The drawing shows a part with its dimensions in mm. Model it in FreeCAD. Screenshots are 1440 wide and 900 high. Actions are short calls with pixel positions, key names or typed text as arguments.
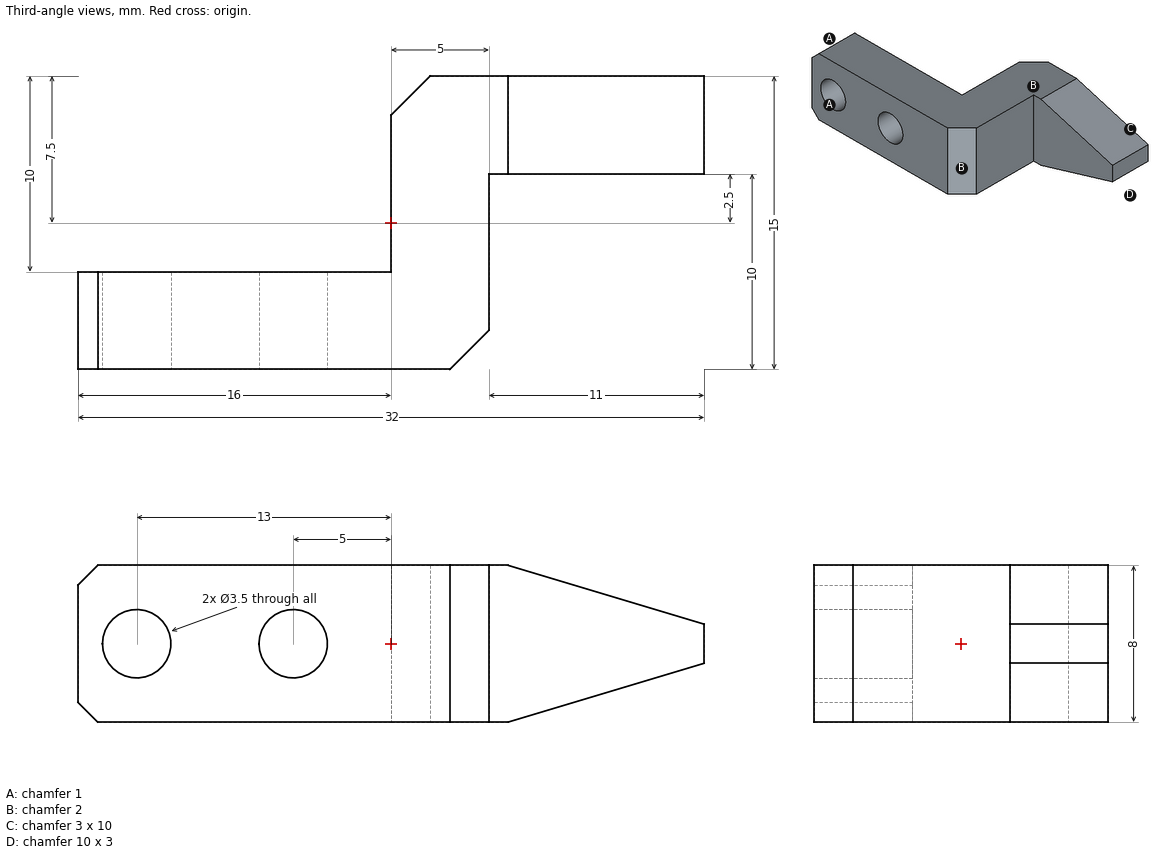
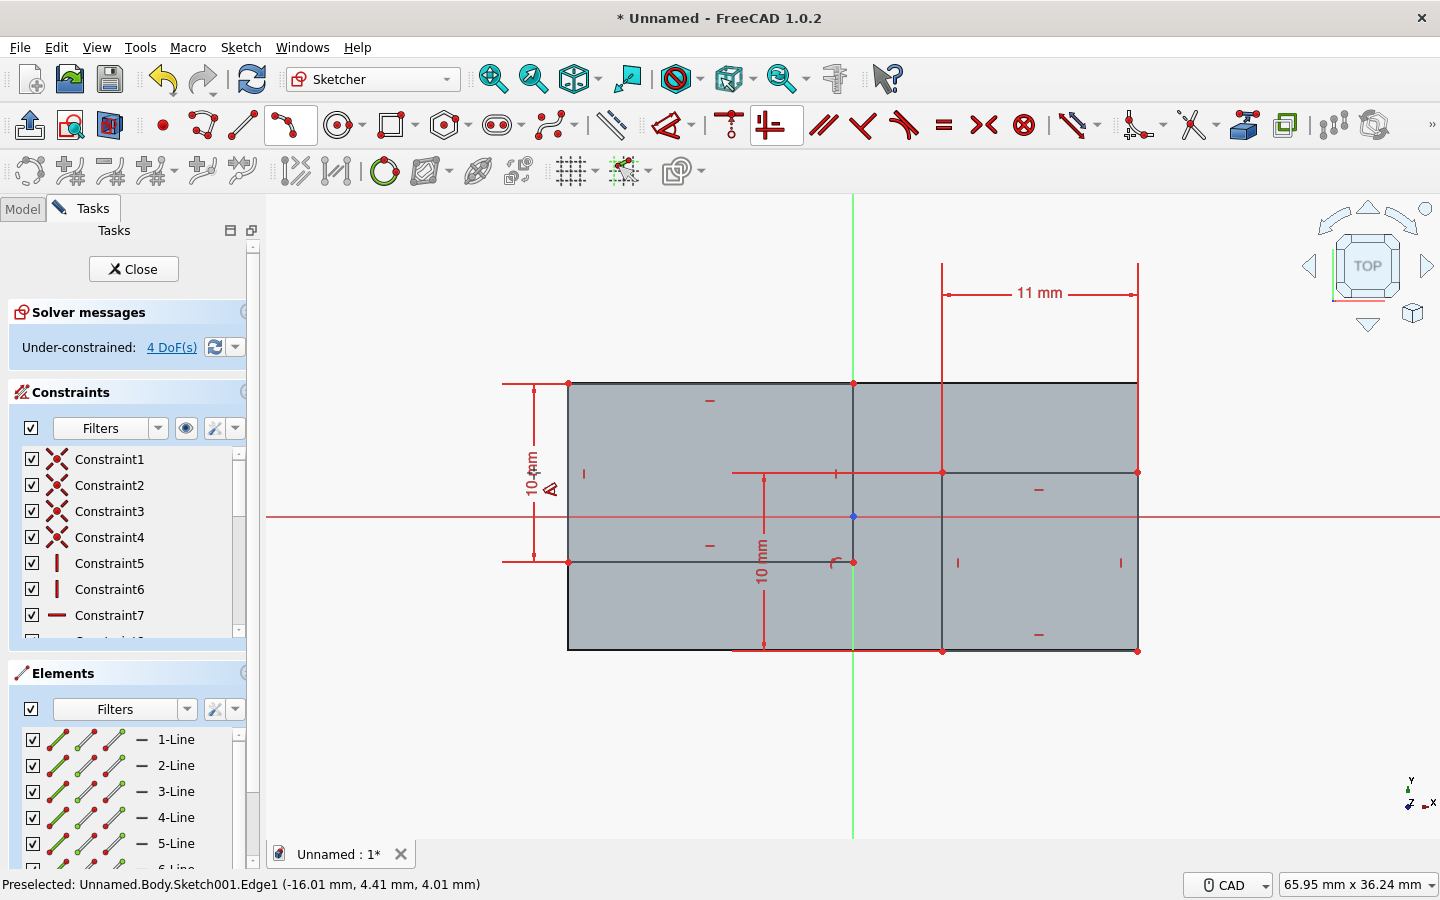
click(654, 562)
click(711, 596)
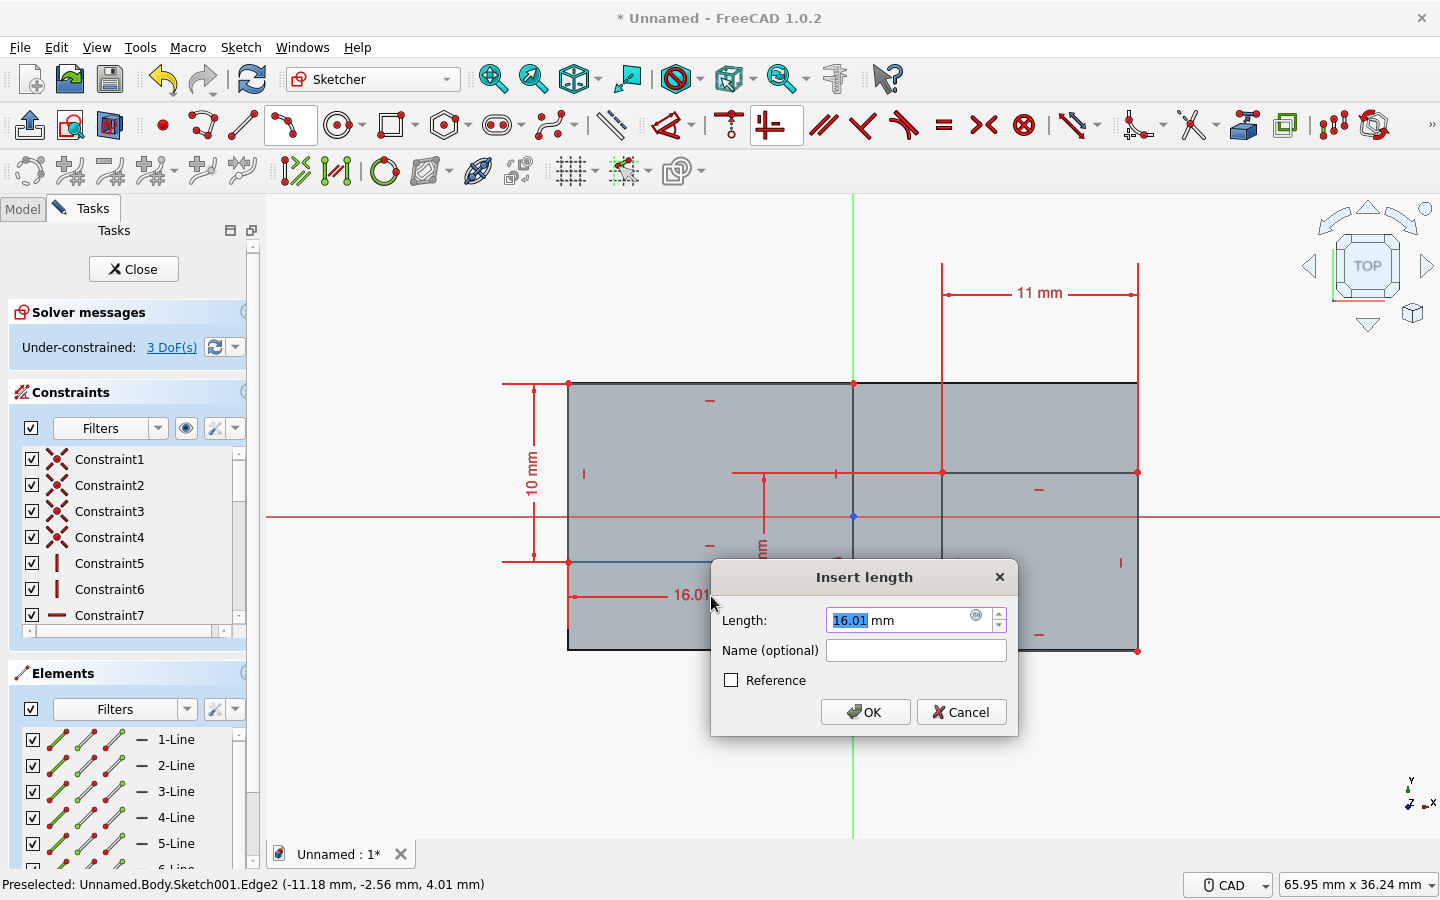
text(16)
key(Return)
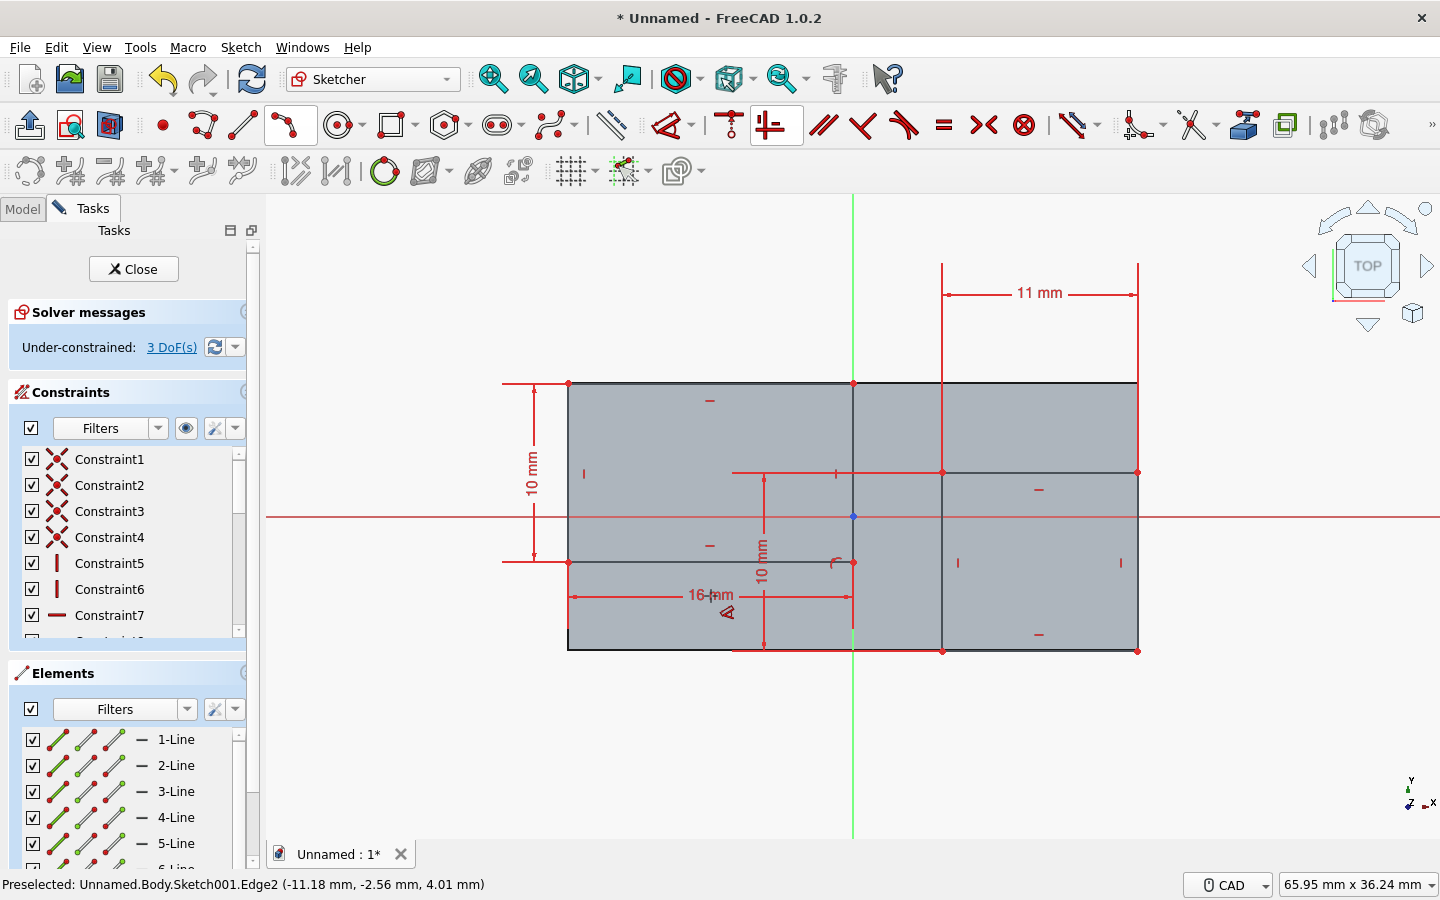
click(942, 473)
click(897, 439)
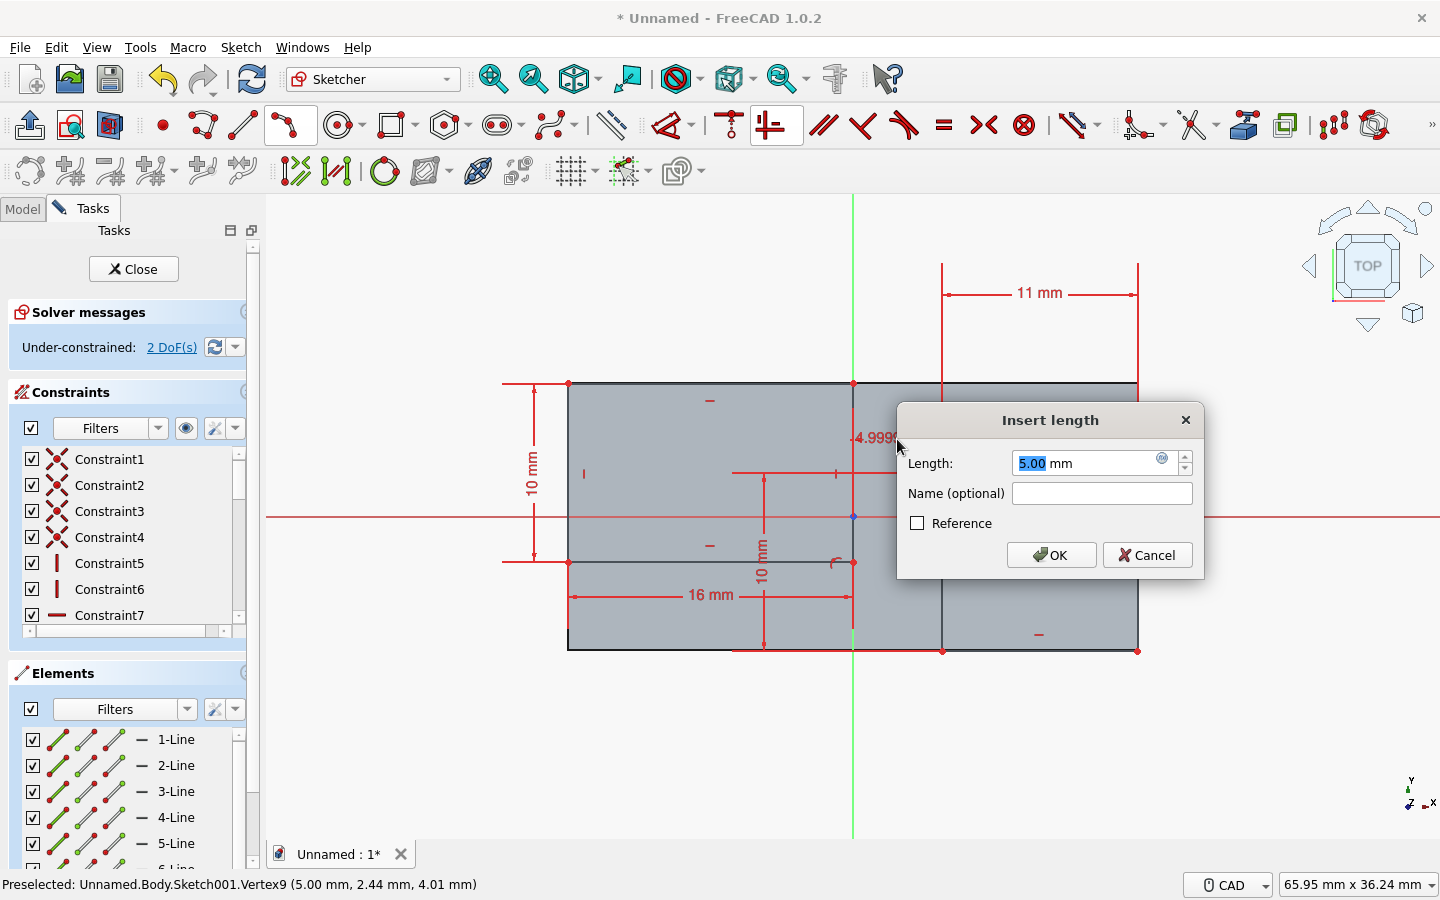
text(5)
key(Return)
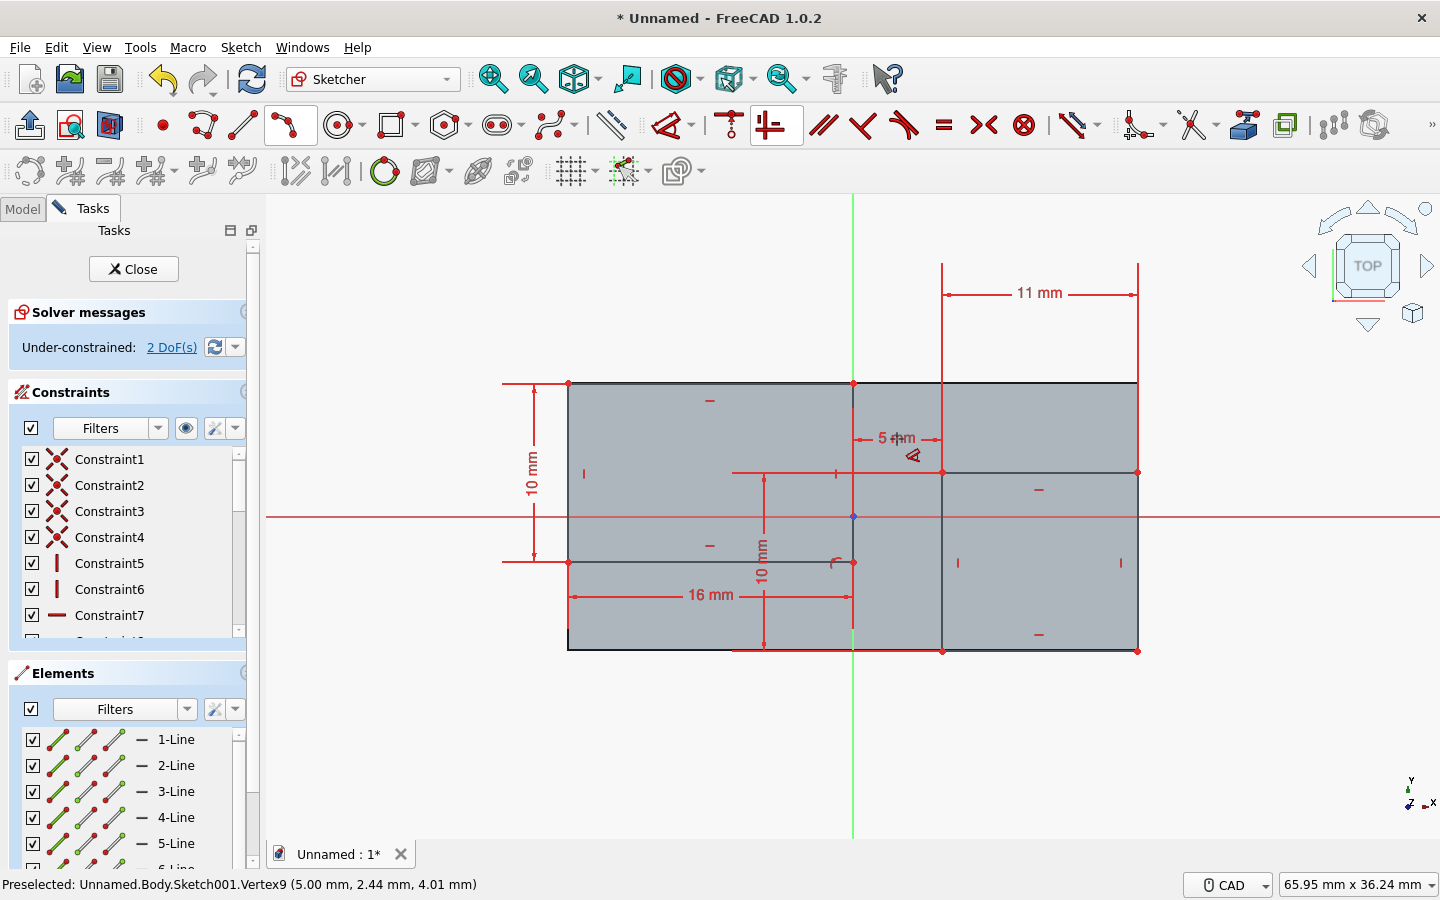
click(568, 384)
click(534, 450)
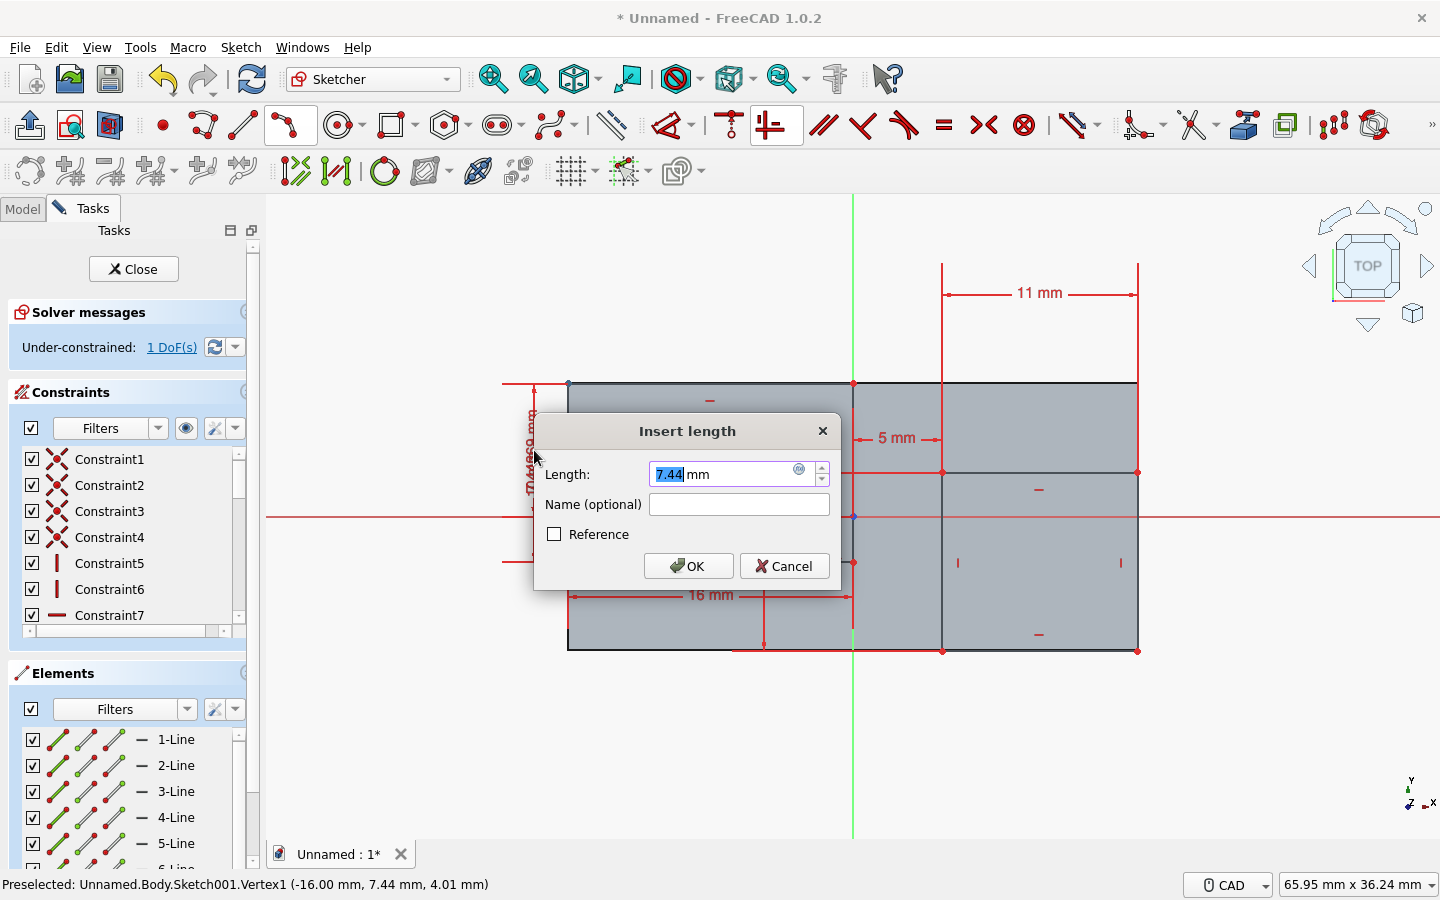
text(7.5)
key(Return)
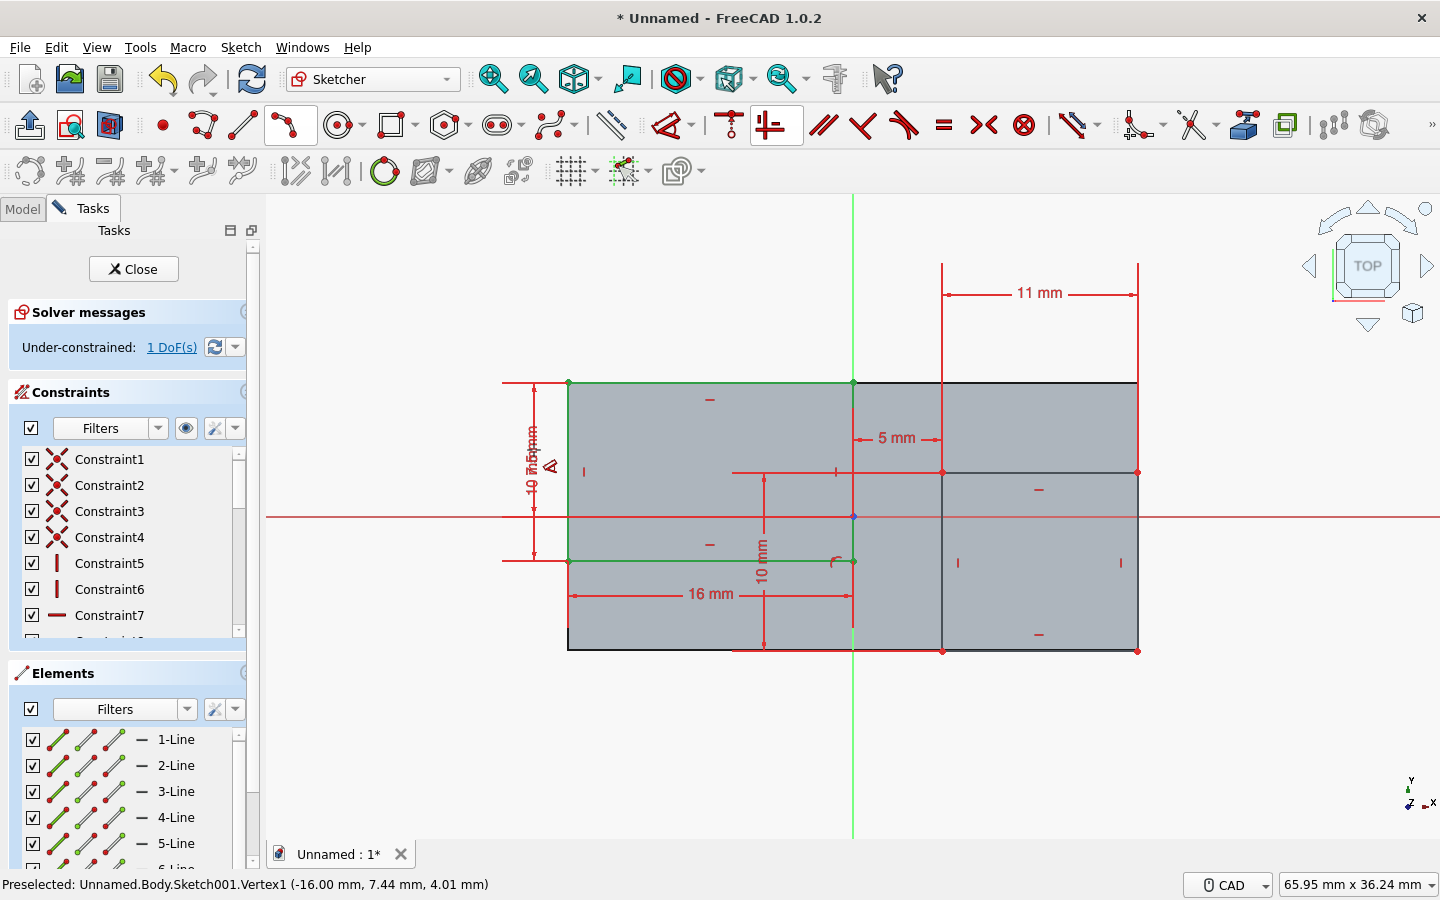
click(942, 473)
click(976, 495)